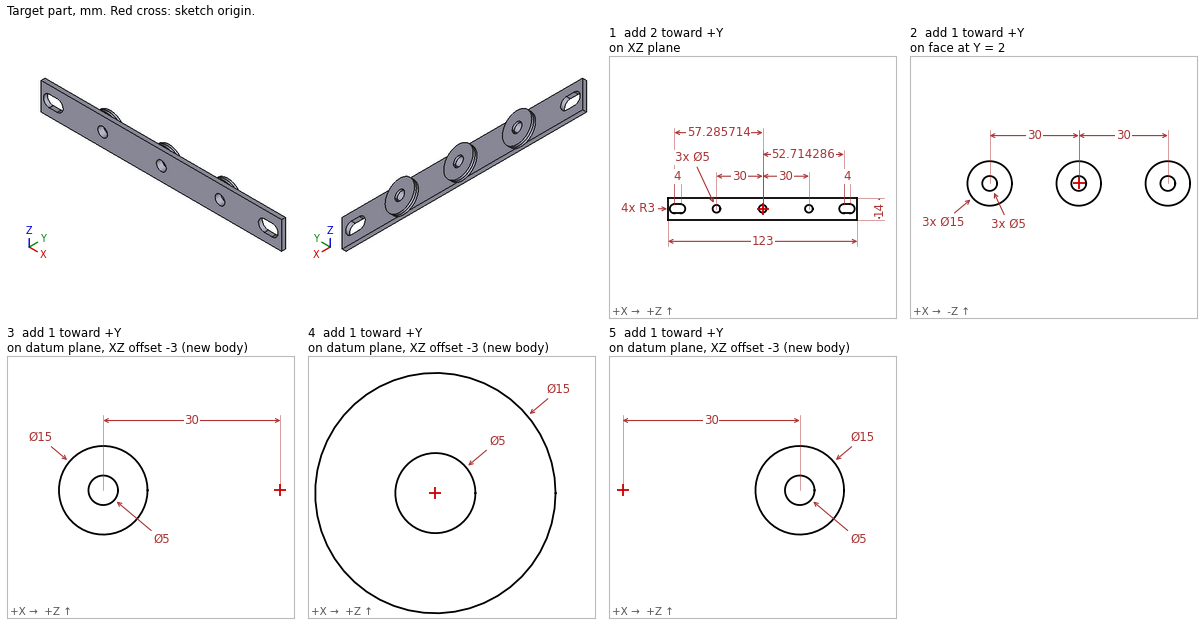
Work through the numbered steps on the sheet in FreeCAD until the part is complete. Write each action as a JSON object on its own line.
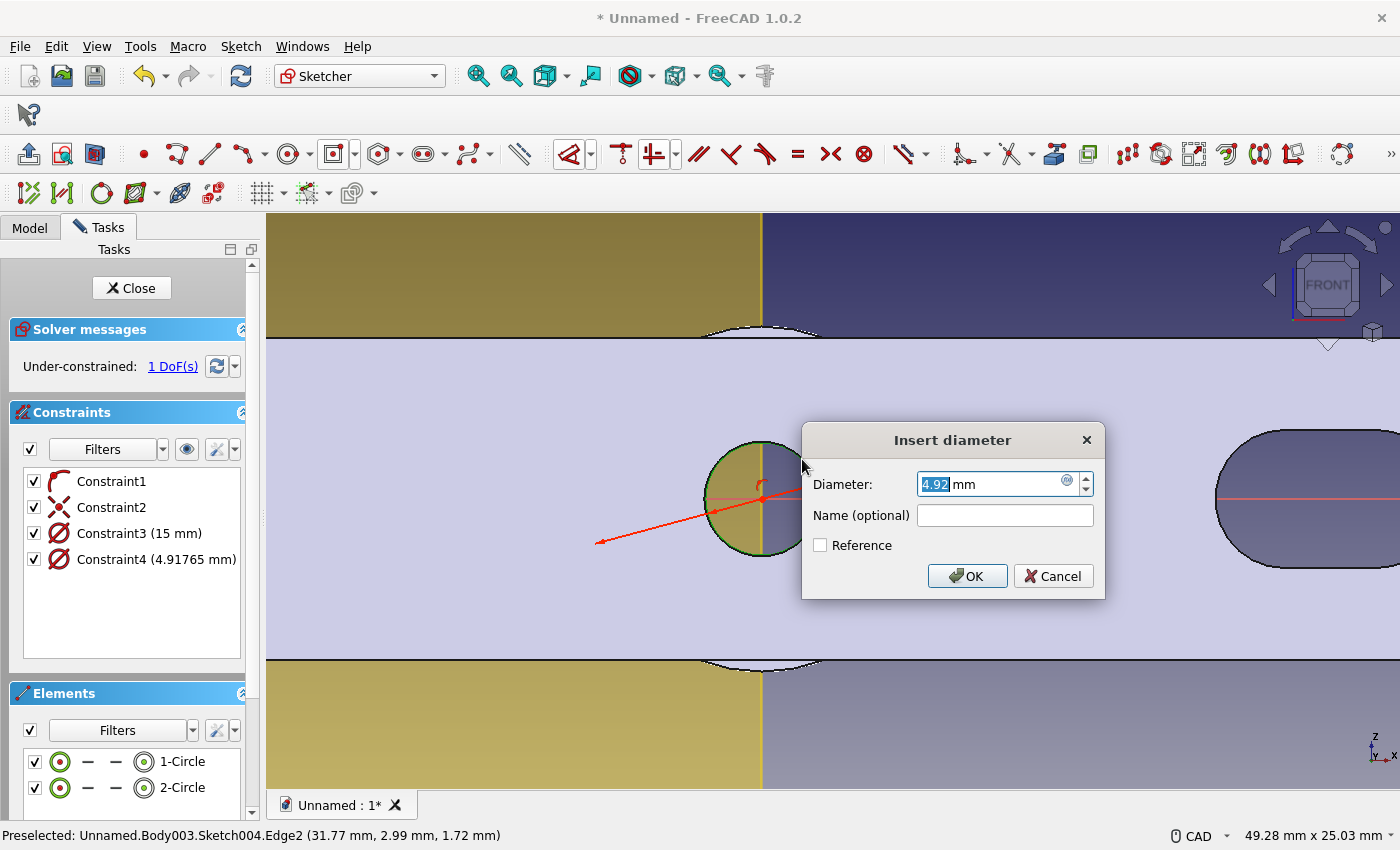
{"action": "type", "text": "5"}
{"action": "key", "text": "Return"}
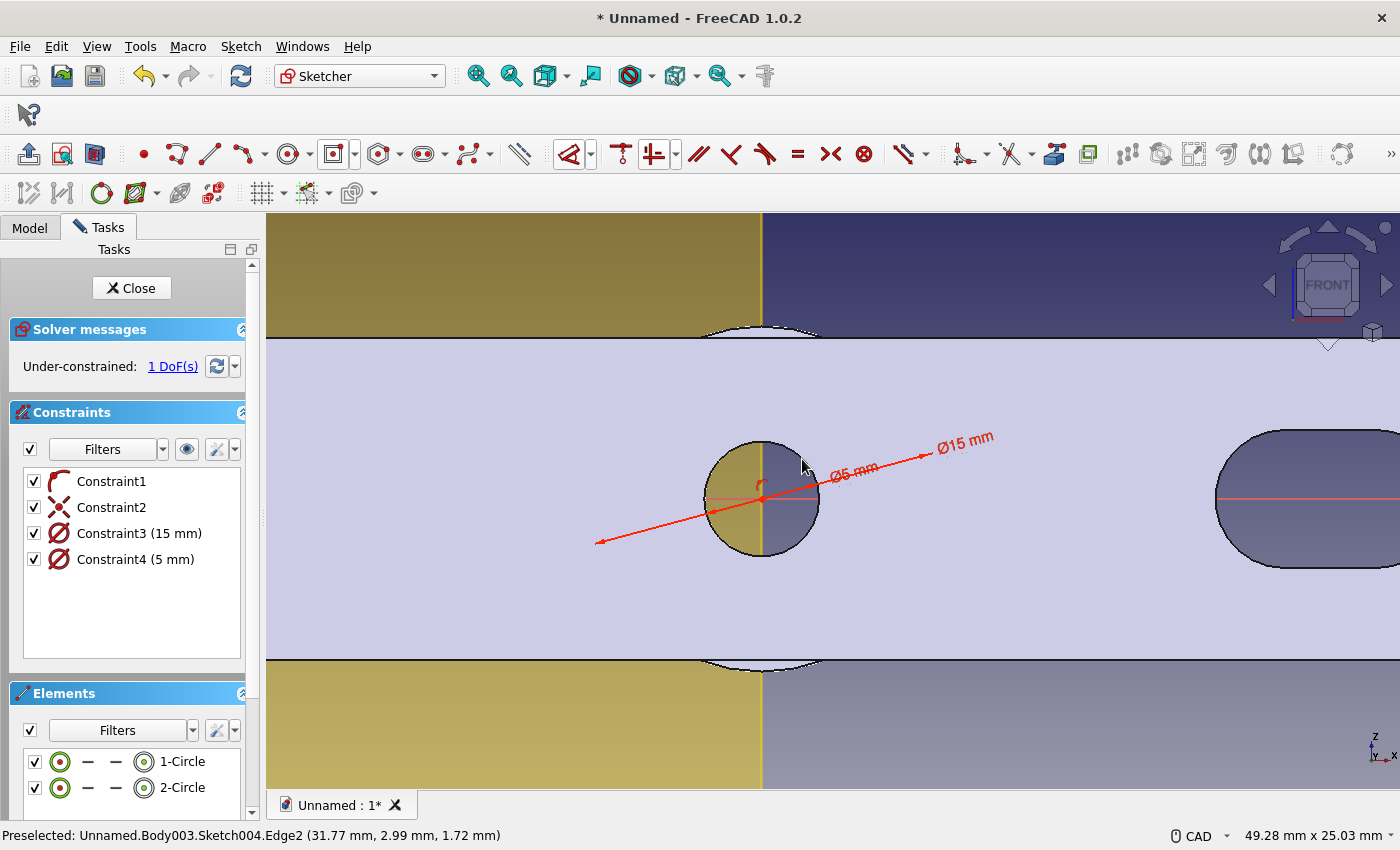
{"action": "left_click", "coordinate": [762, 499]}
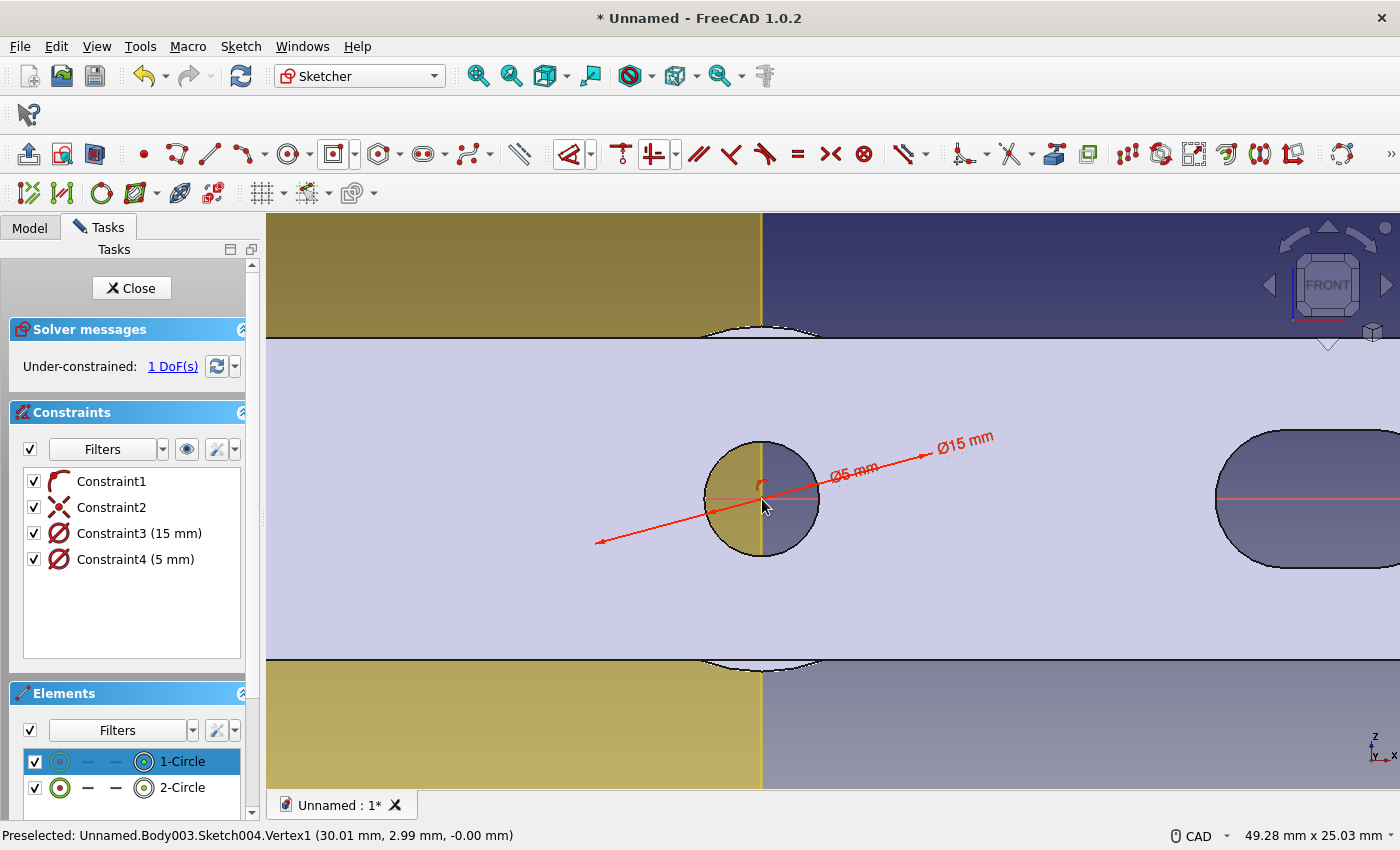
{"action": "left_click", "coordinate": [590, 154]}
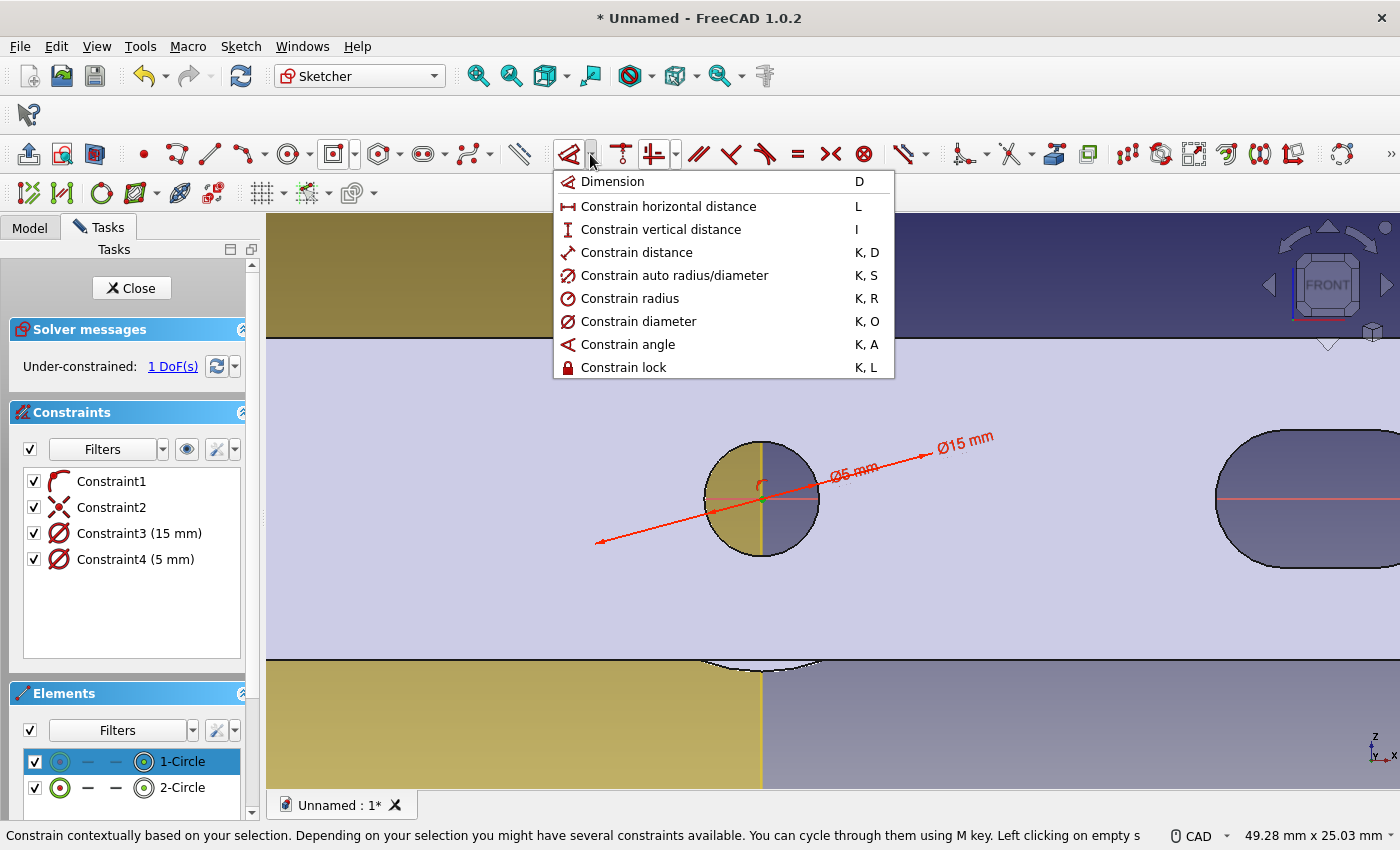
{"action": "left_click", "coordinate": [724, 206]}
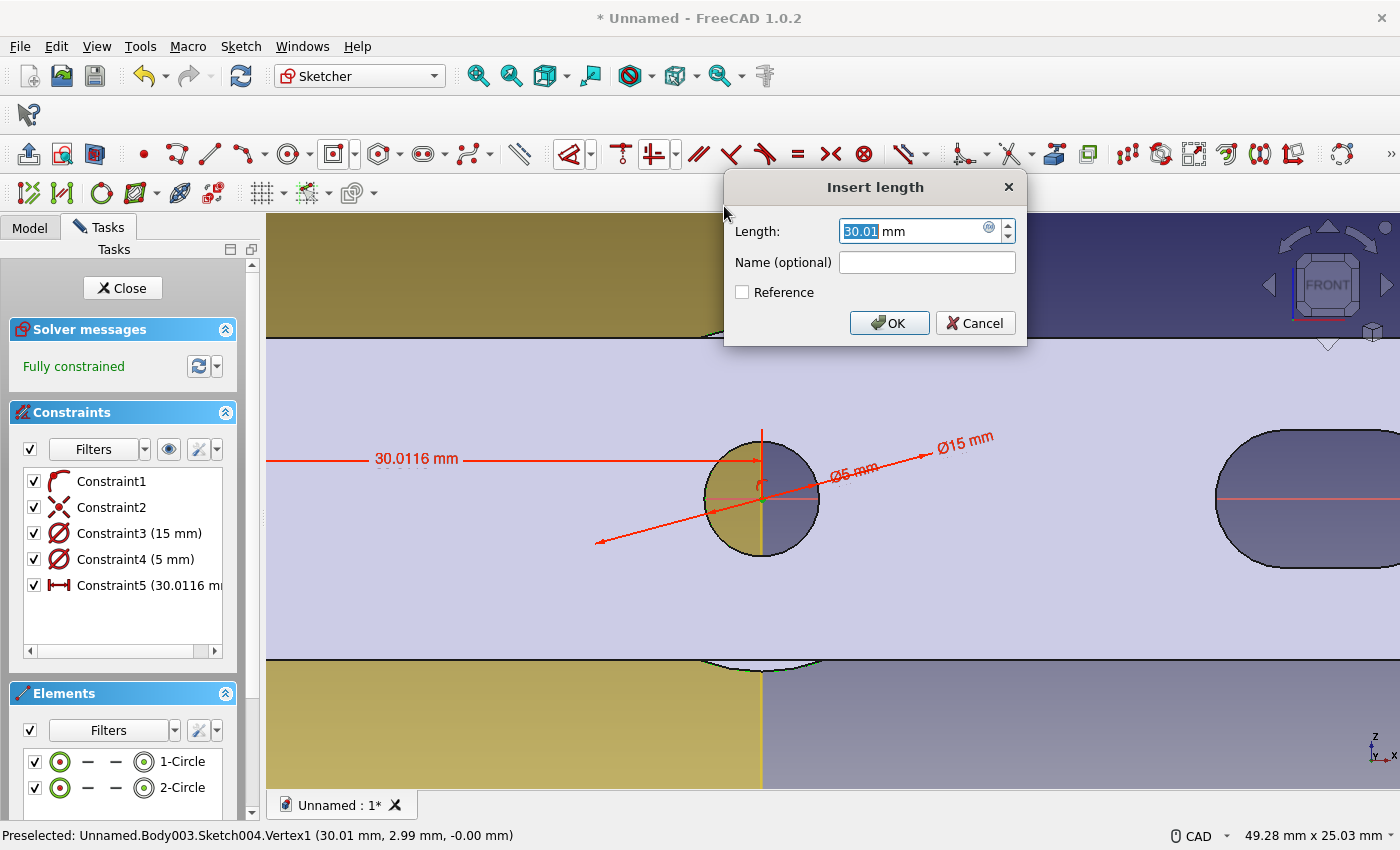
{"action": "type", "text": "30"}
{"action": "key", "text": "Return"}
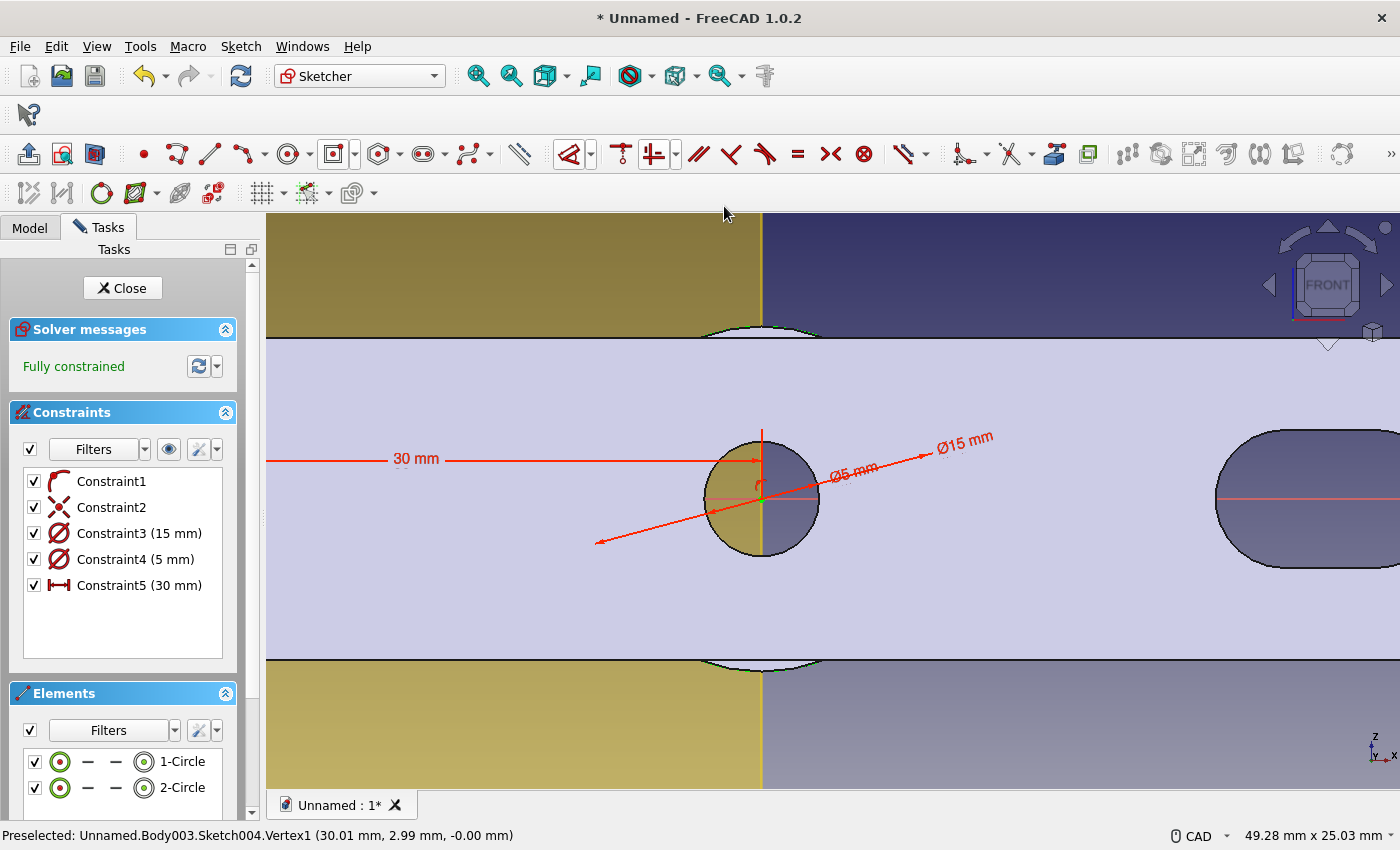
{"action": "left_click", "coordinate": [123, 288]}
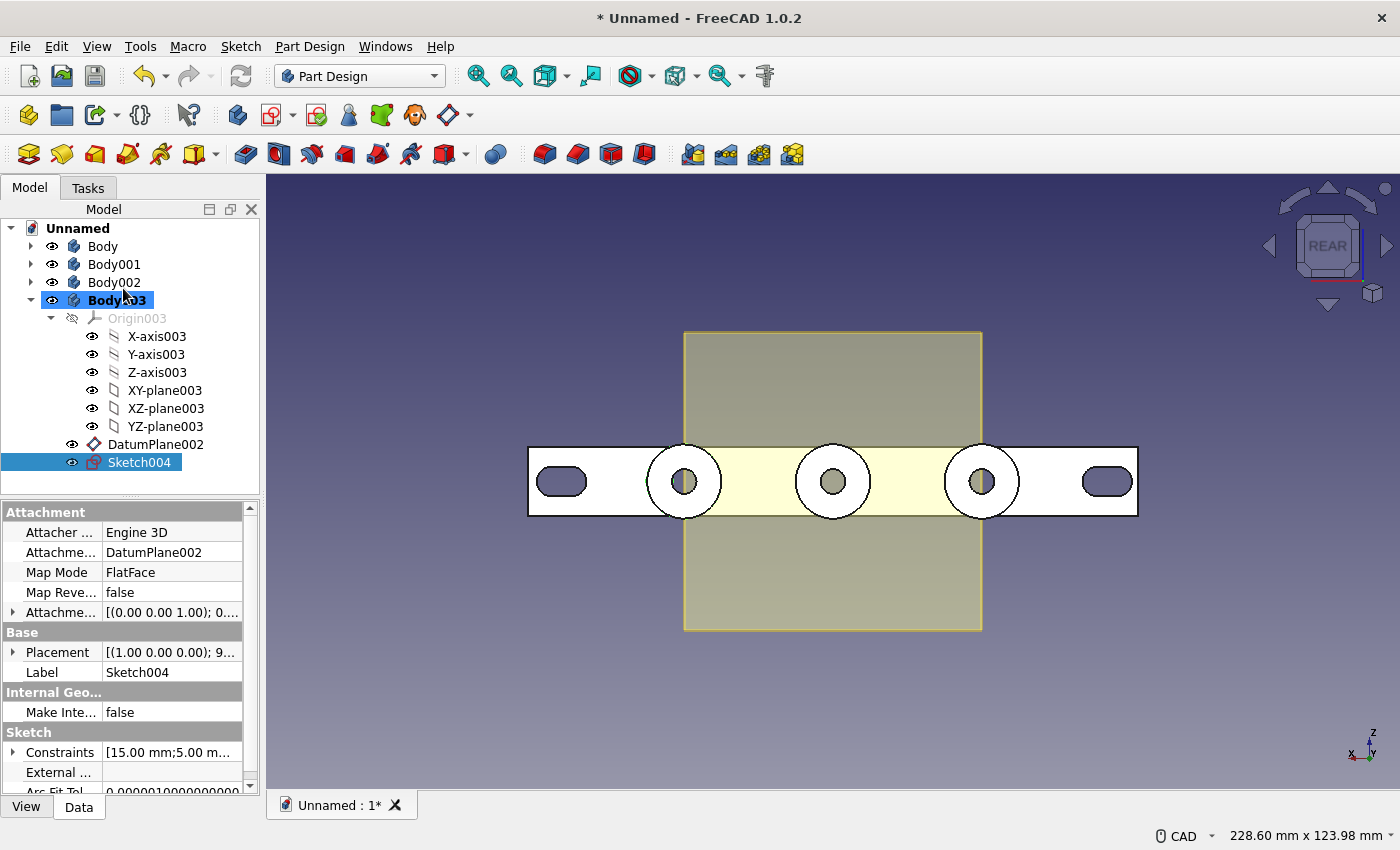
{"action": "left_click", "coordinate": [29, 154]}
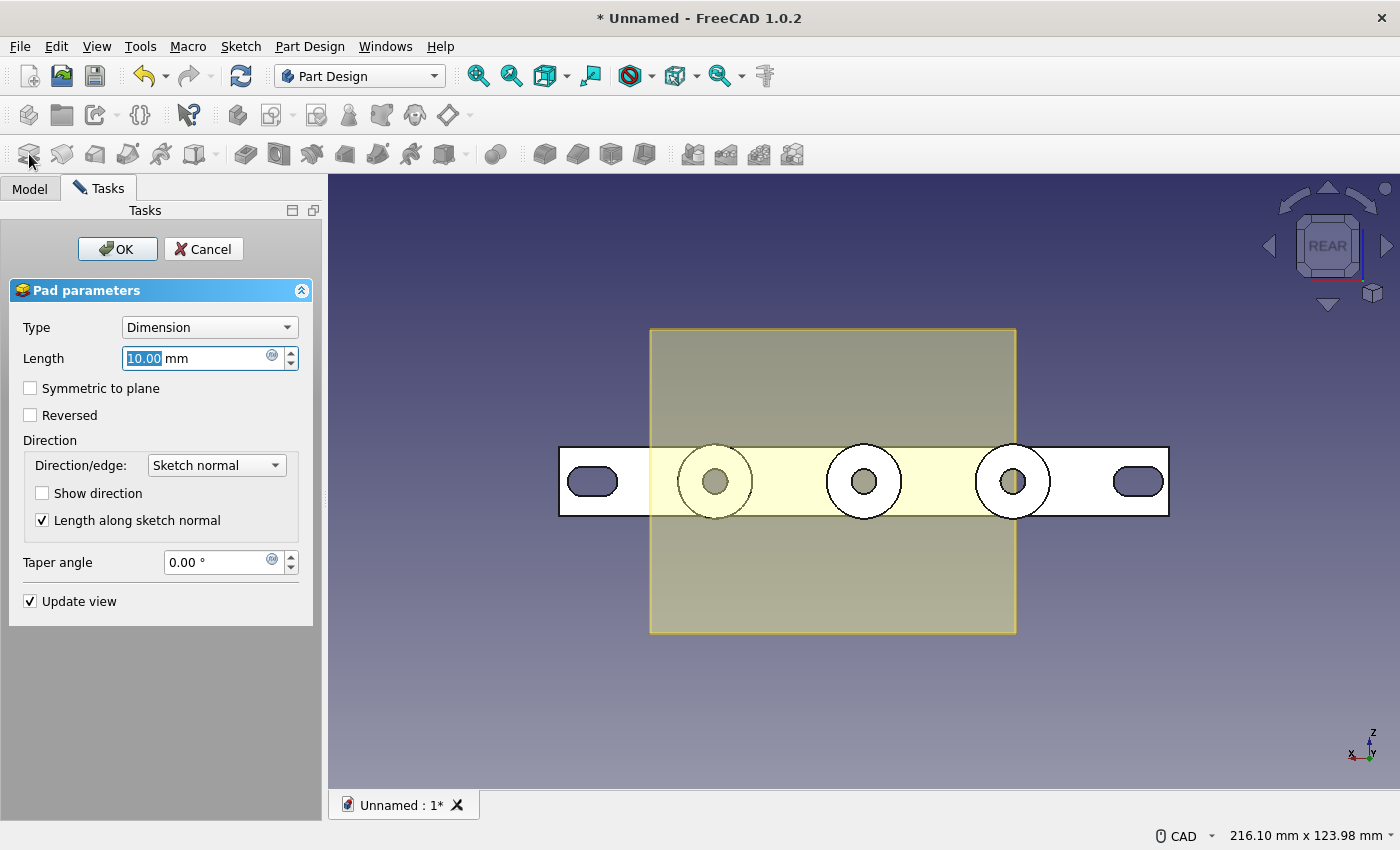
{"action": "type", "text": "1"}
{"action": "key", "text": "Tab"}